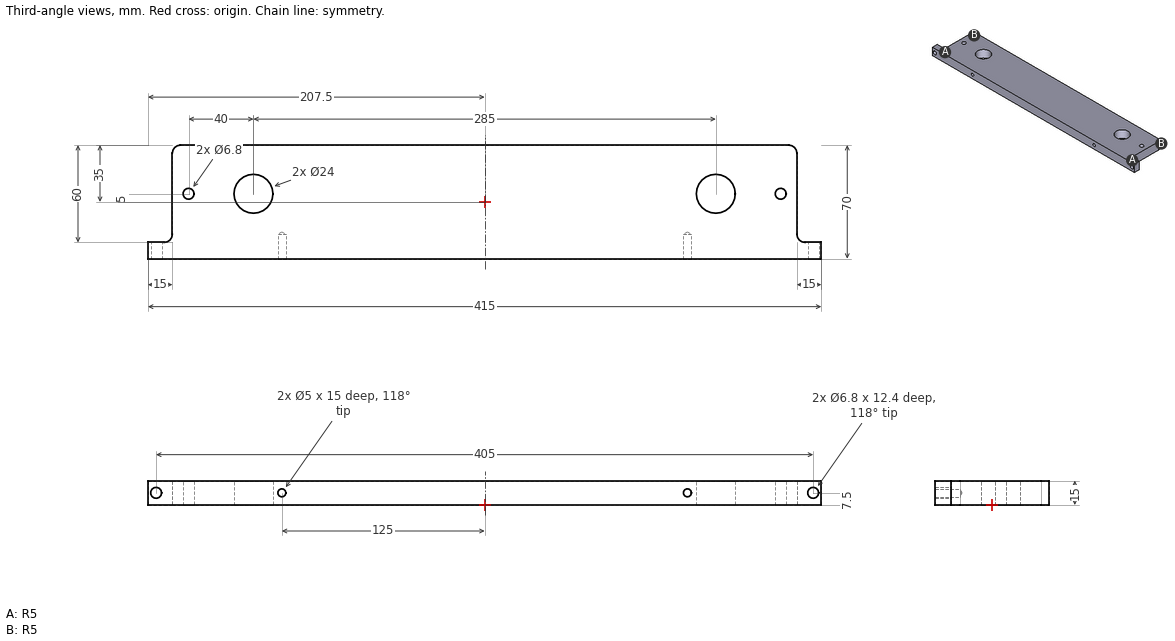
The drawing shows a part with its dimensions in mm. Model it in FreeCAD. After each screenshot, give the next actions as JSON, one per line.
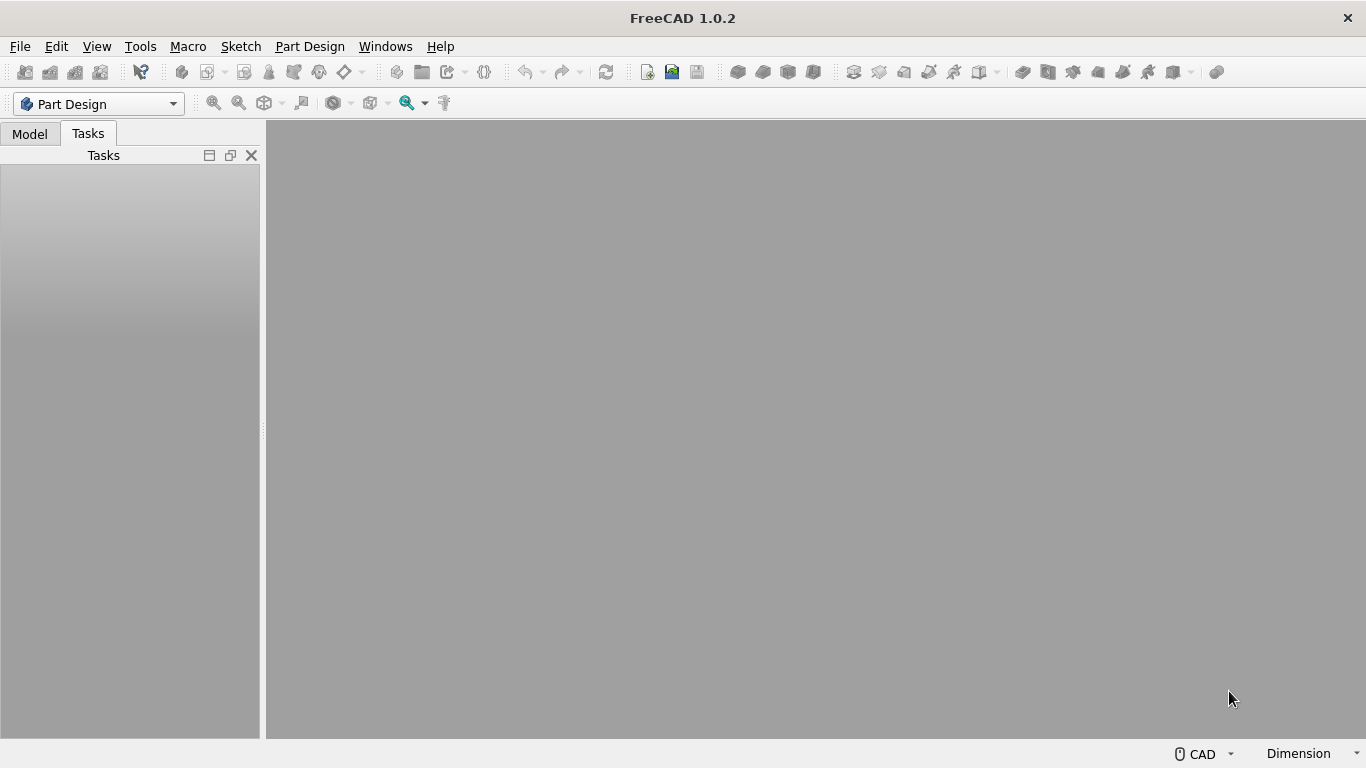
{"action": "key", "text": "ctrl+n"}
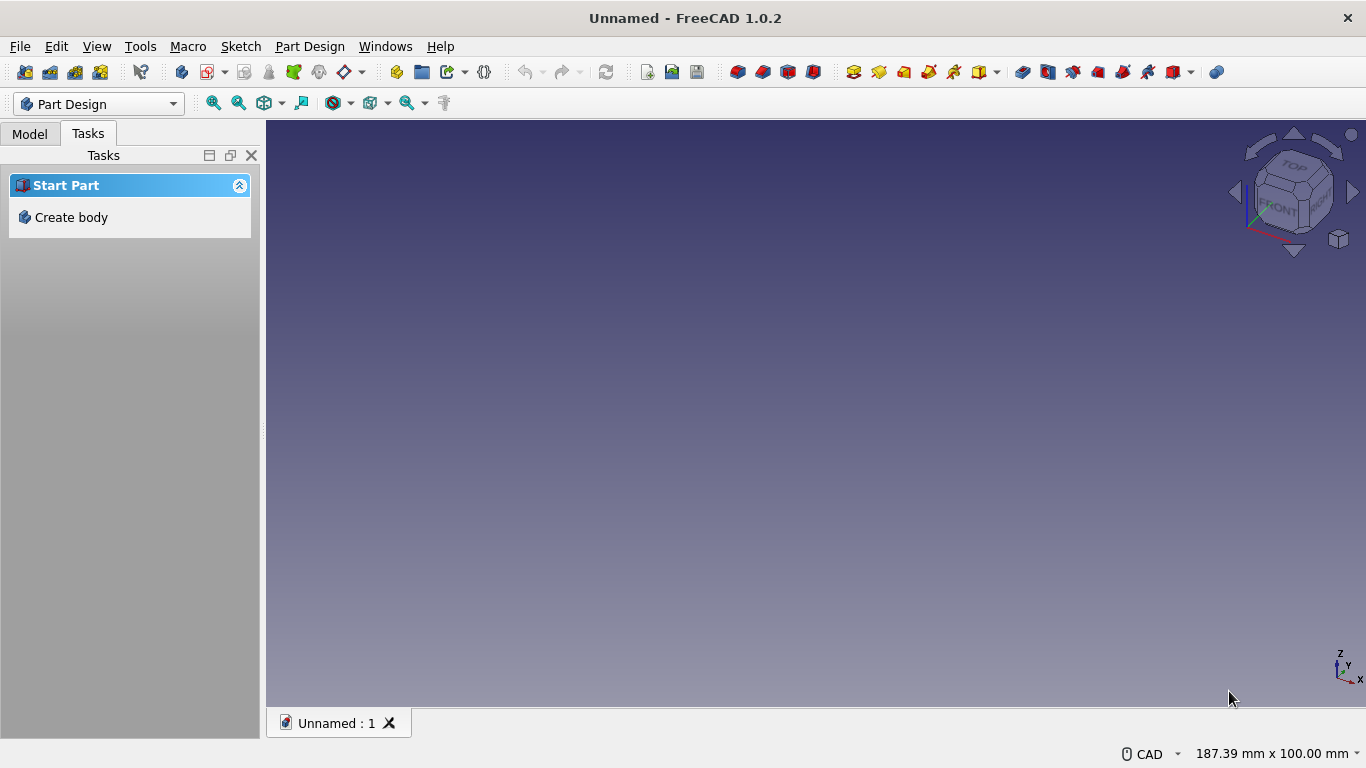
{"action": "left_click", "coordinate": [206, 72]}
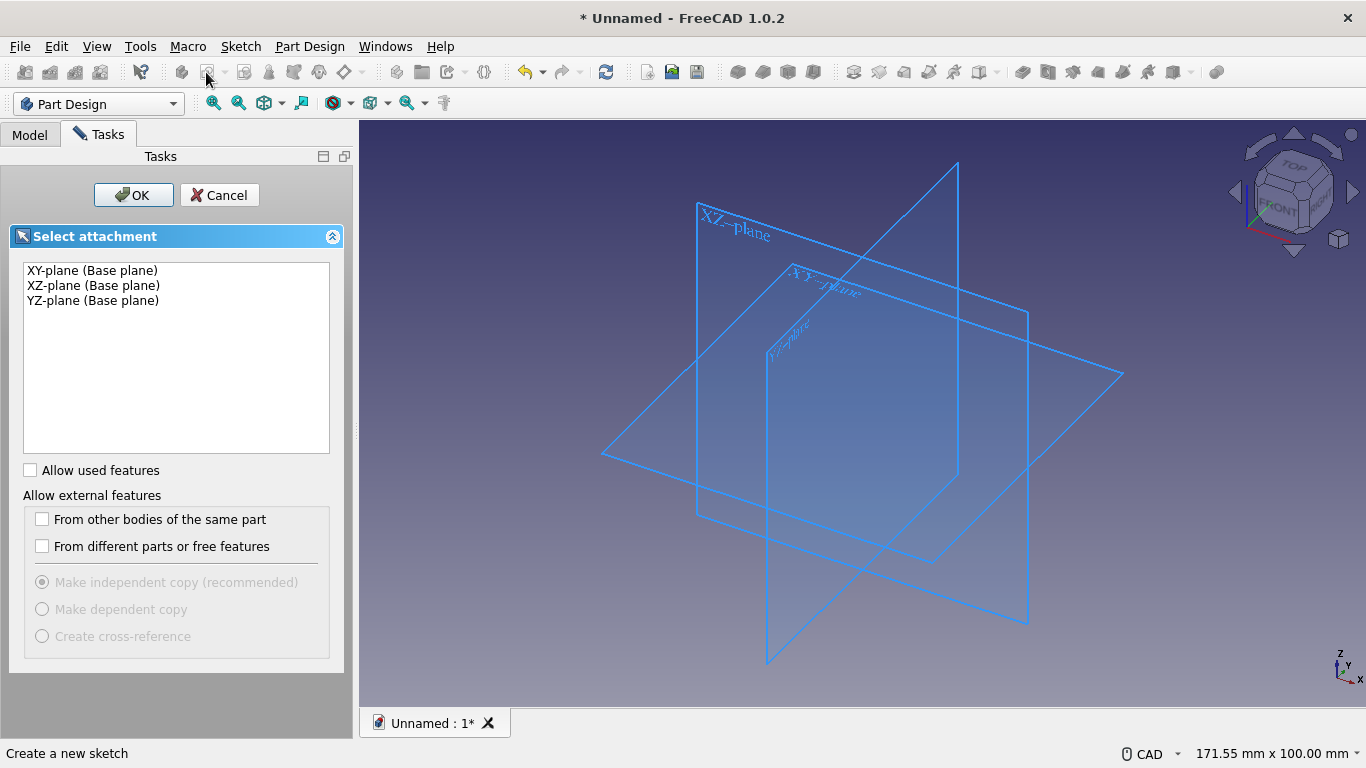
{"action": "left_click", "coordinate": [84, 270]}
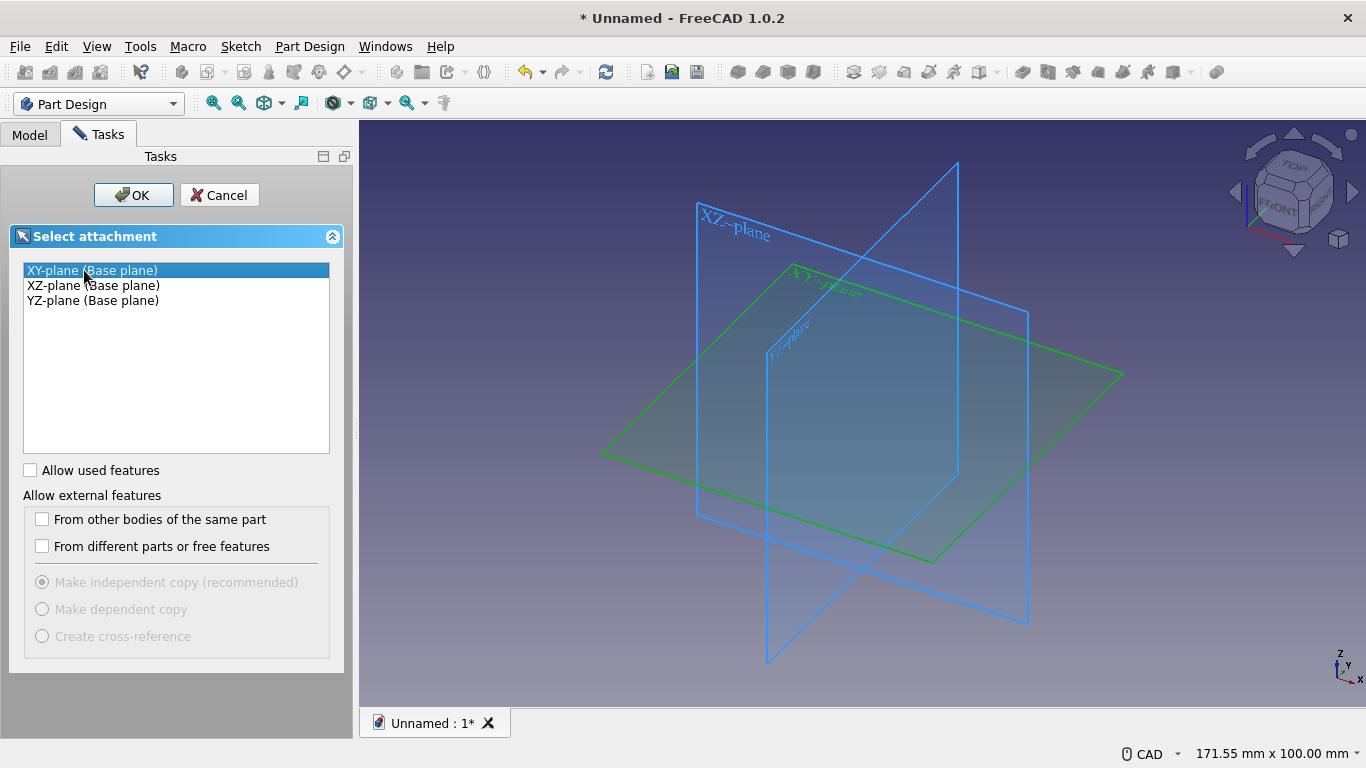
{"action": "left_click", "coordinate": [134, 195]}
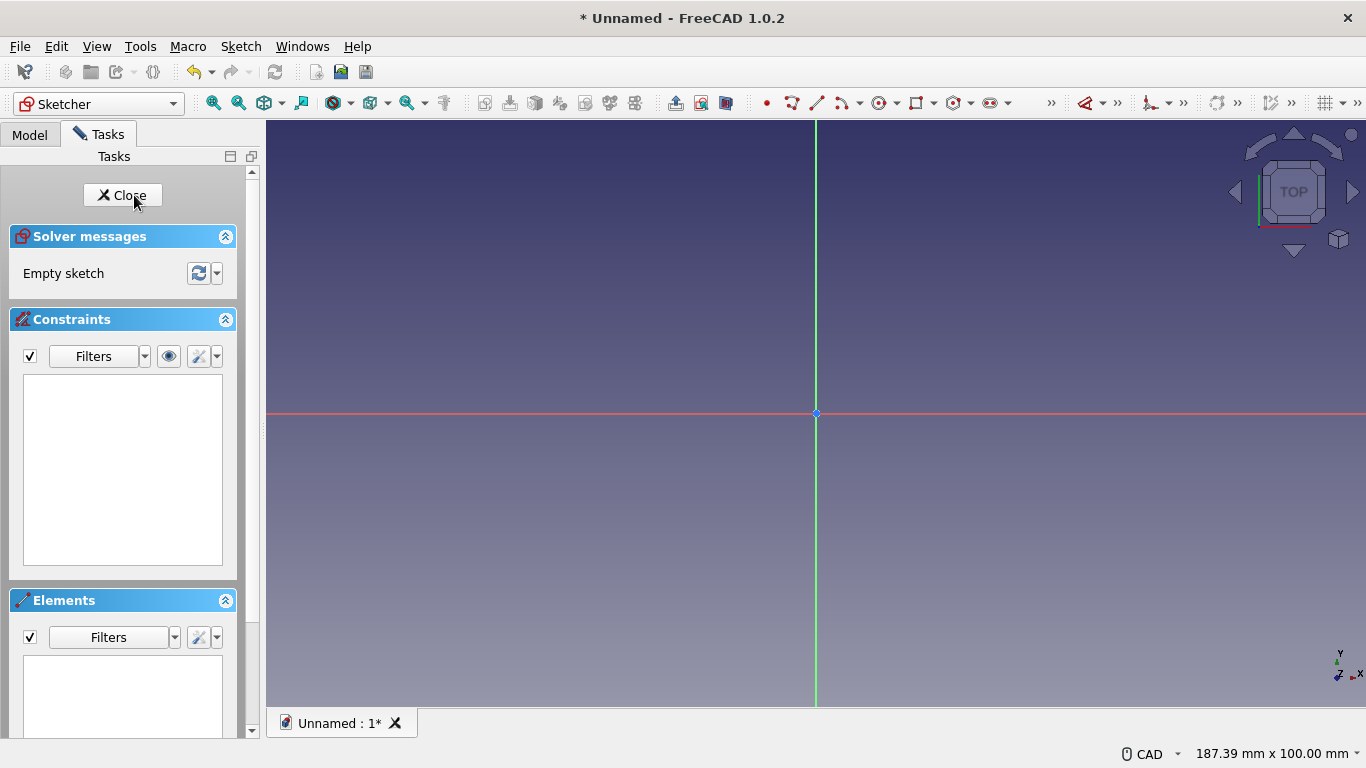
{"action": "scroll", "coordinate": [725, 414], "scroll_direction": "down", "scroll_amount": 7}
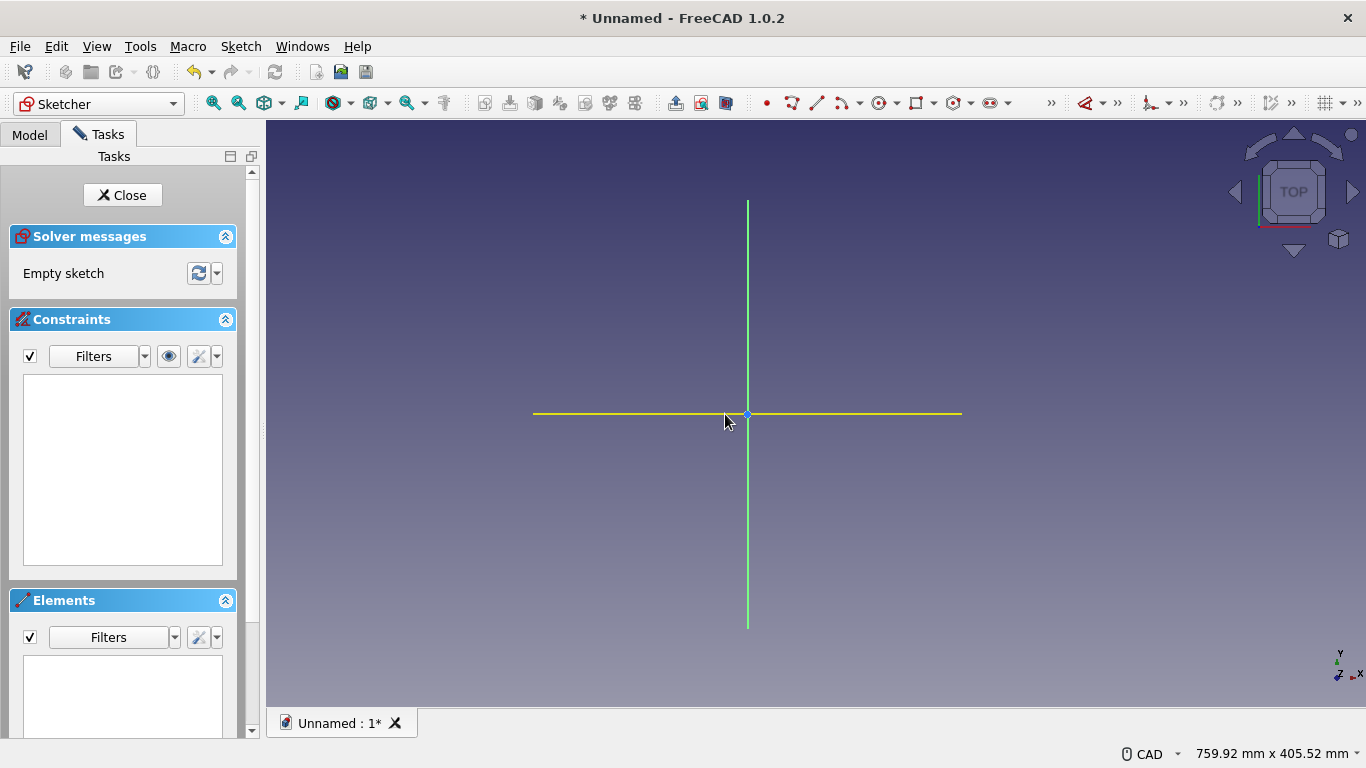
{"action": "key", "text": "g v"}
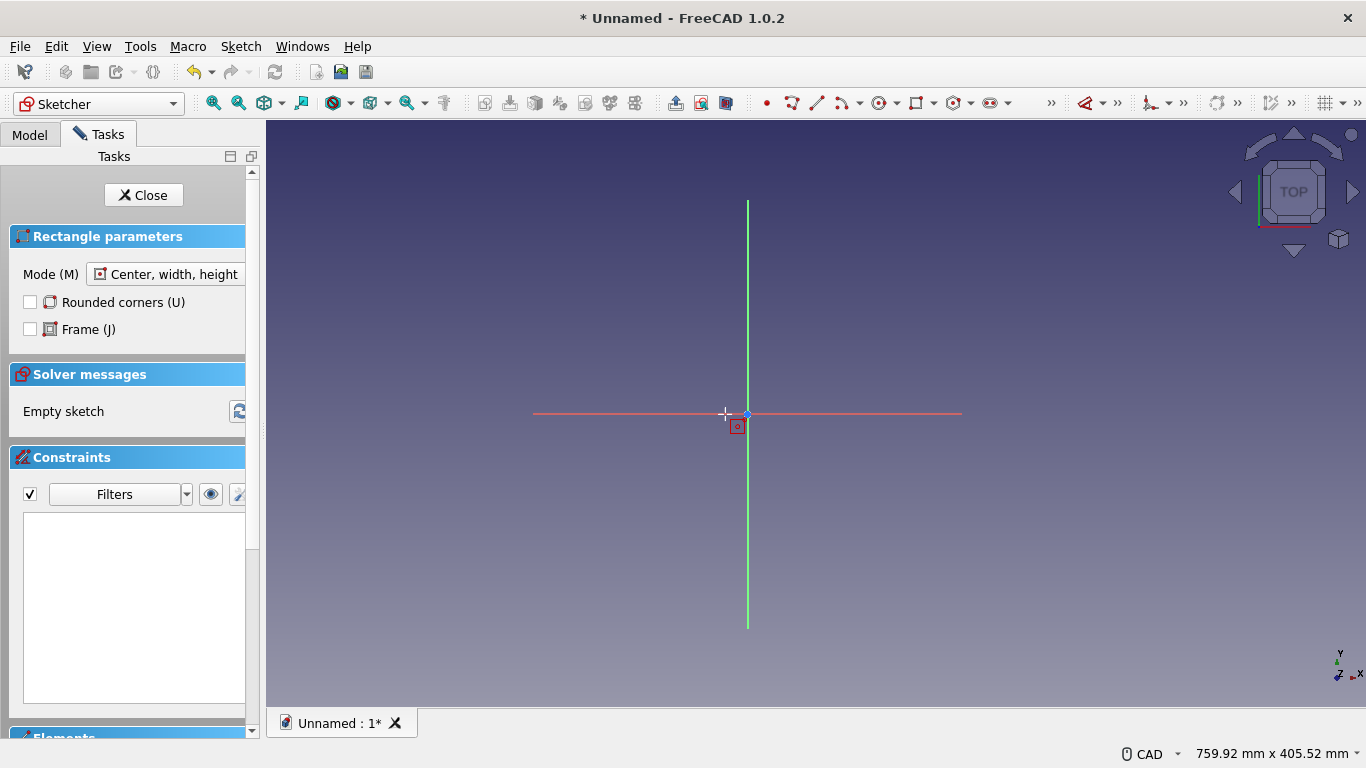
{"action": "left_click", "coordinate": [748, 414]}
{"action": "mouse_move", "coordinate": [1048, 364]}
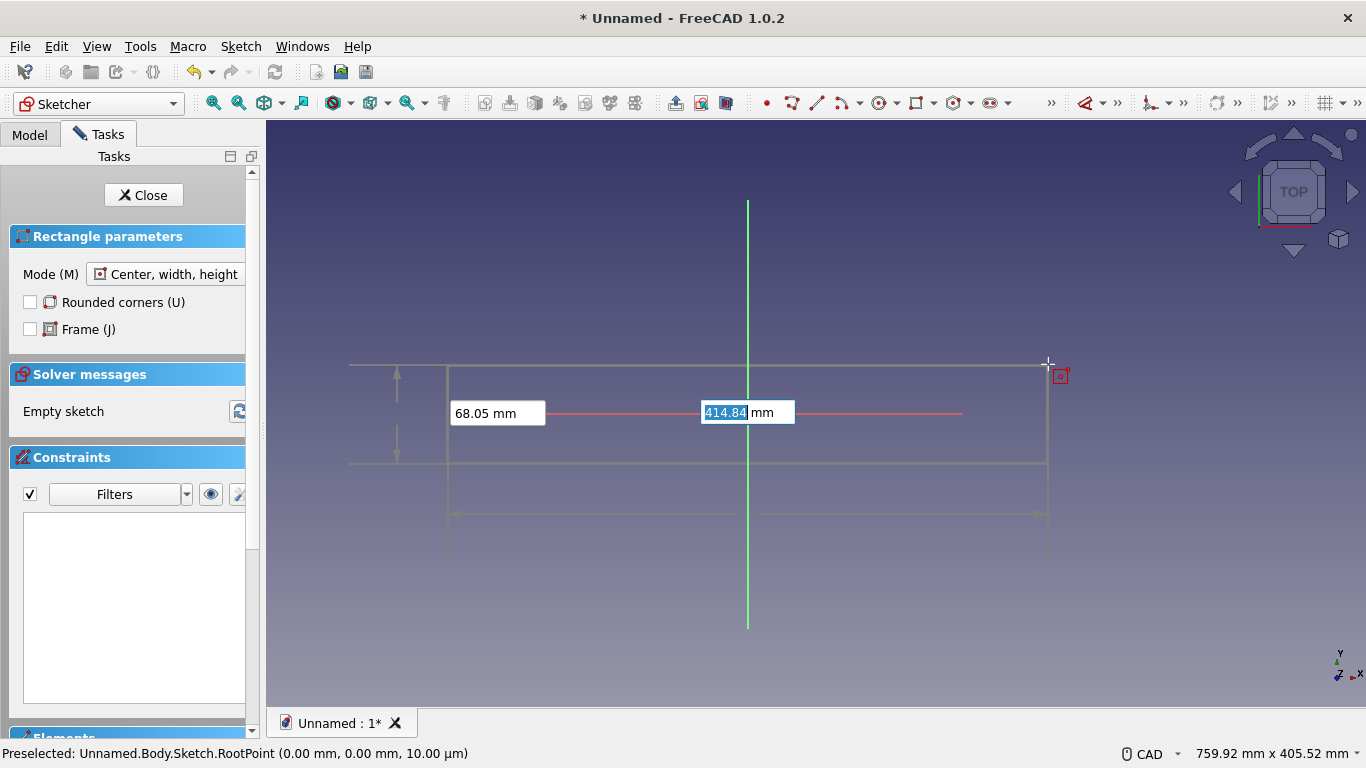
{"action": "type", "text": "415"}
{"action": "key", "text": "Tab"}
{"action": "type", "text": "70"}
{"action": "key", "text": "Return"}
{"action": "key", "text": "Escape"}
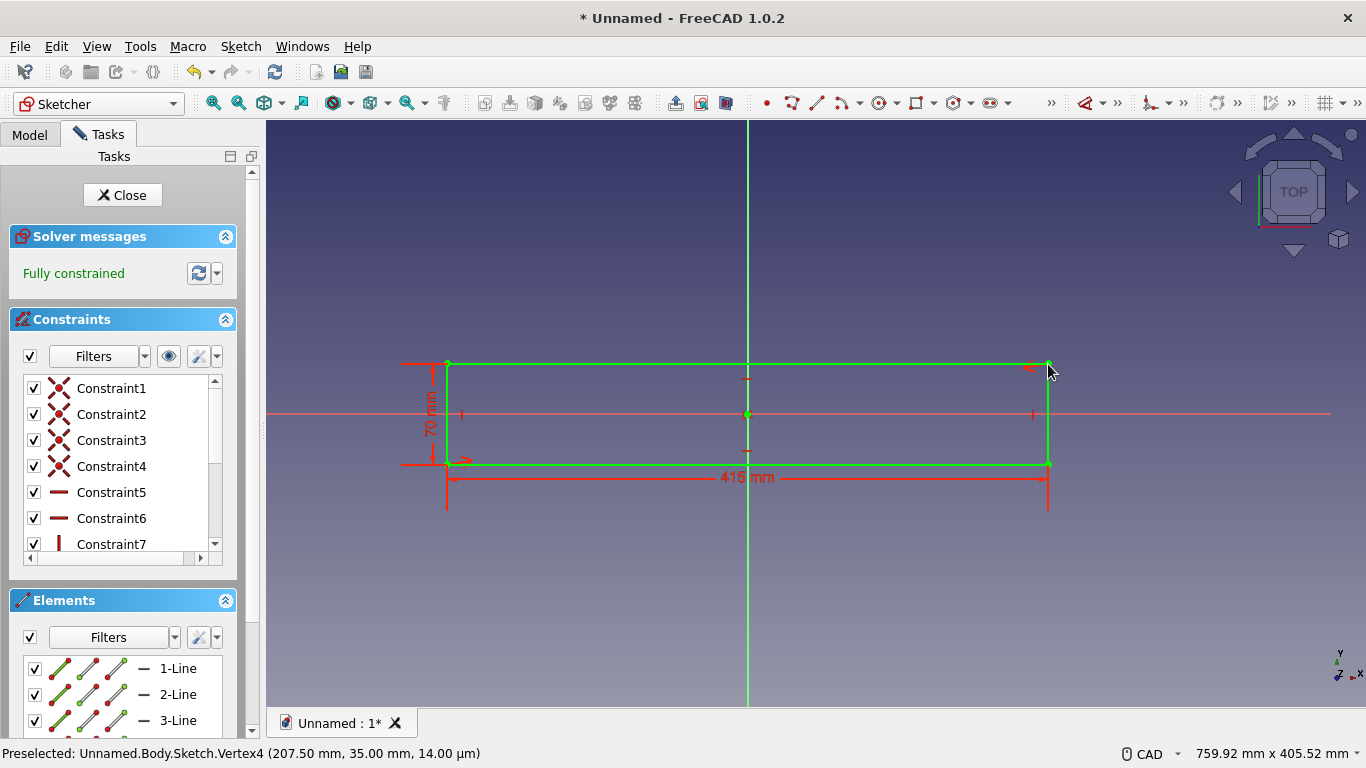
{"action": "left_click", "coordinate": [123, 195]}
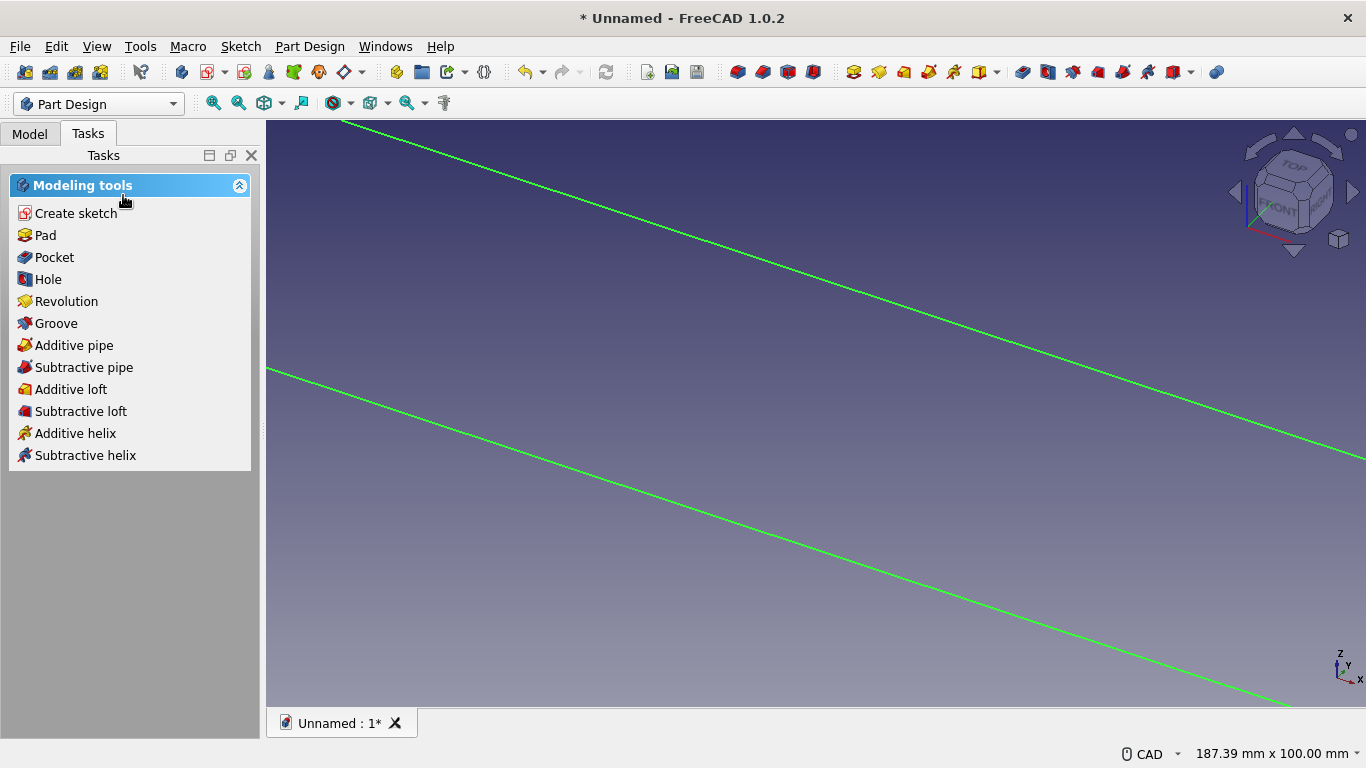
{"action": "left_click", "coordinate": [854, 72]}